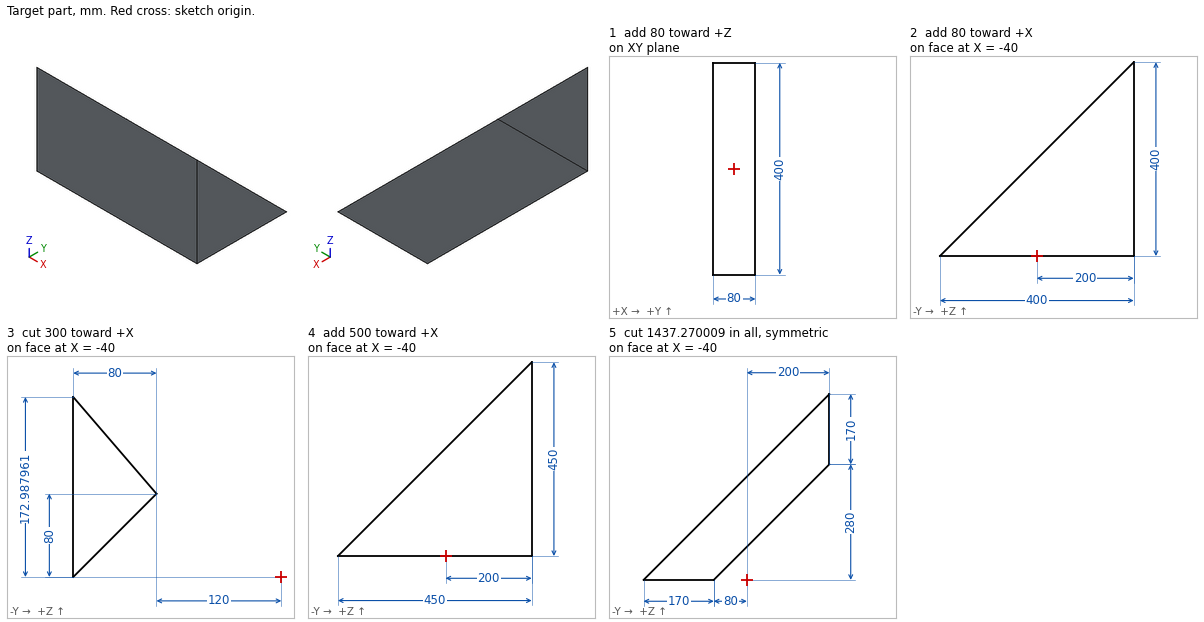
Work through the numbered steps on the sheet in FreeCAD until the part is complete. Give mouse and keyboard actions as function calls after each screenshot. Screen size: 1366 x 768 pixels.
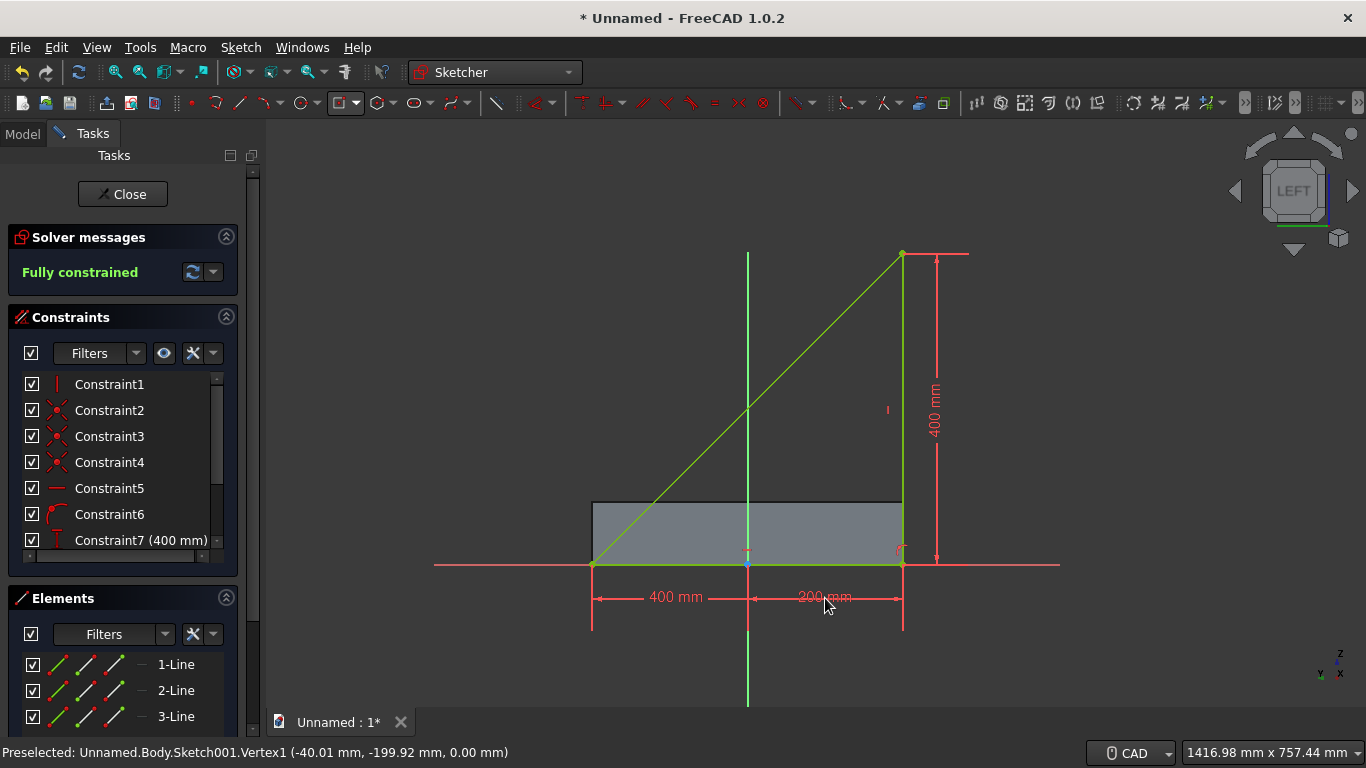
click(123, 194)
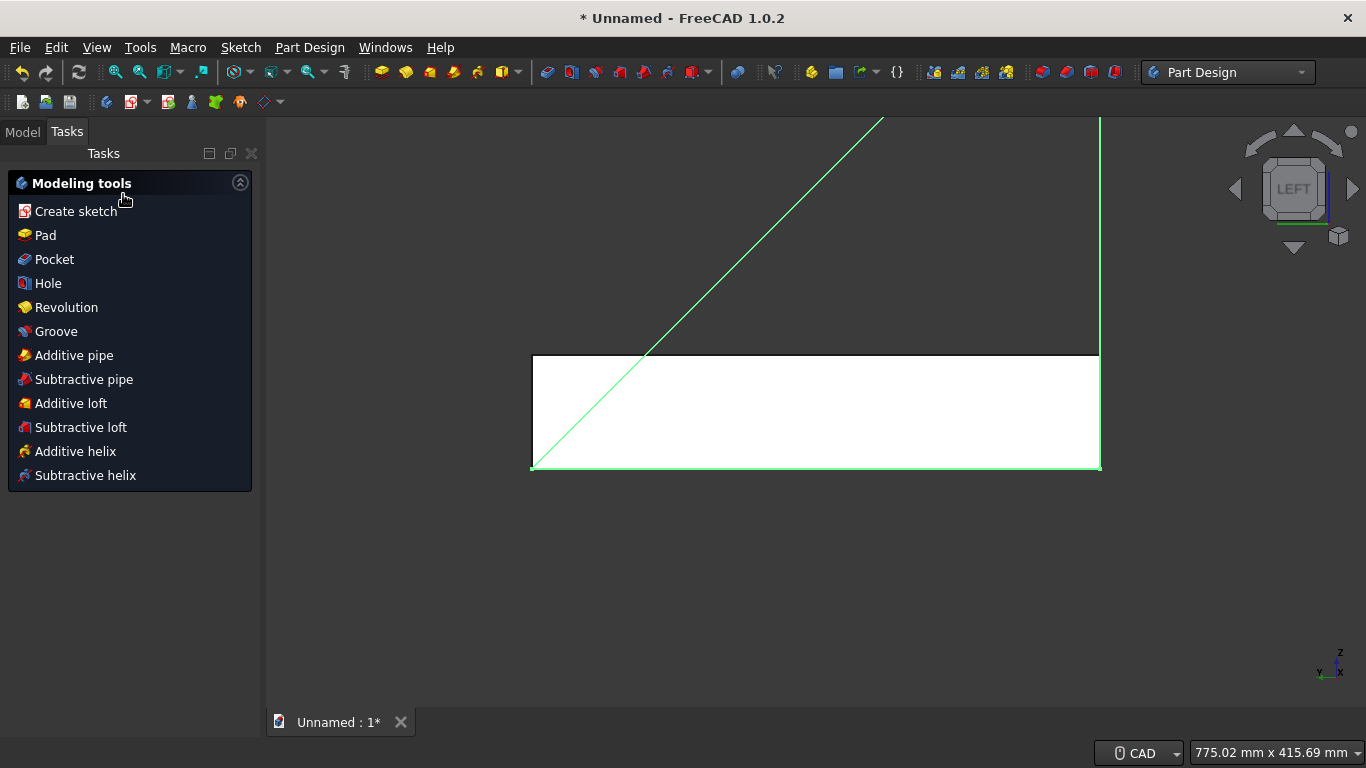
click(382, 72)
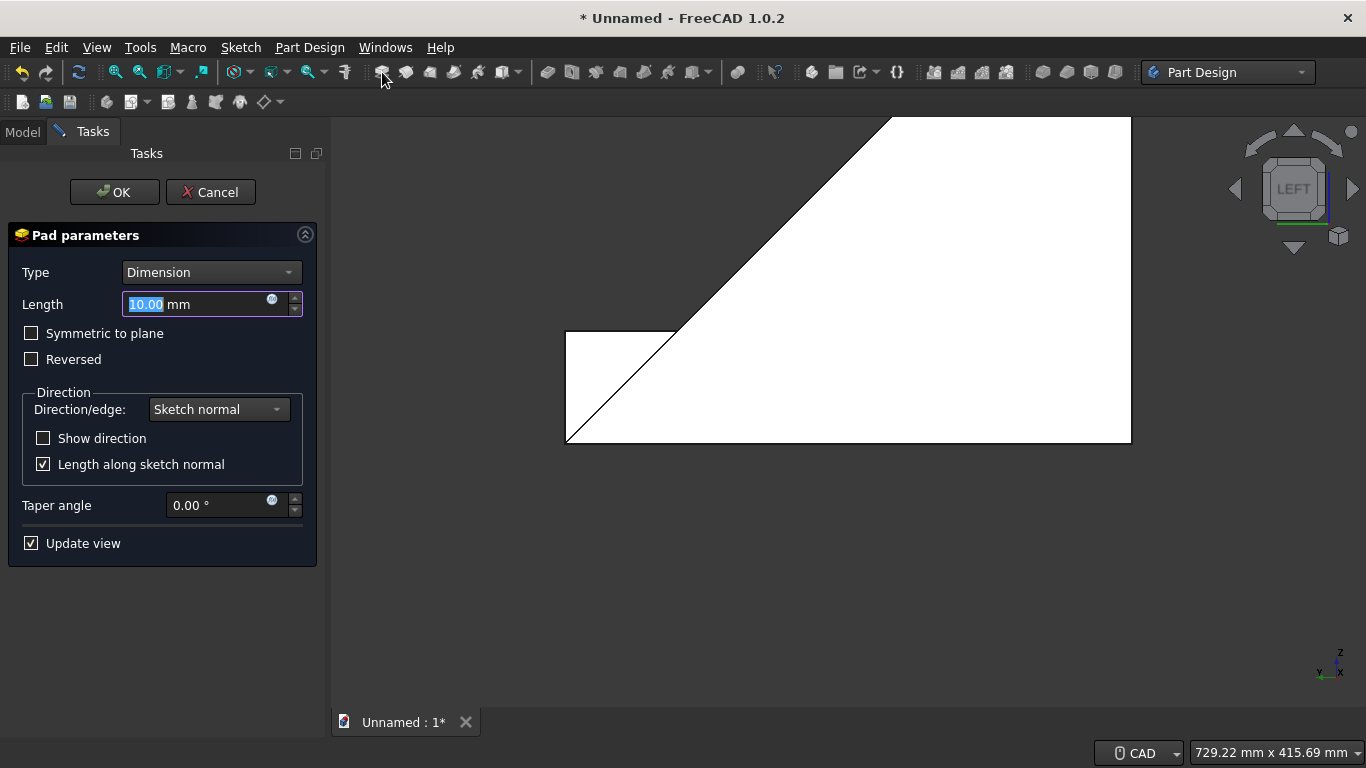
text(80)
key(Tab)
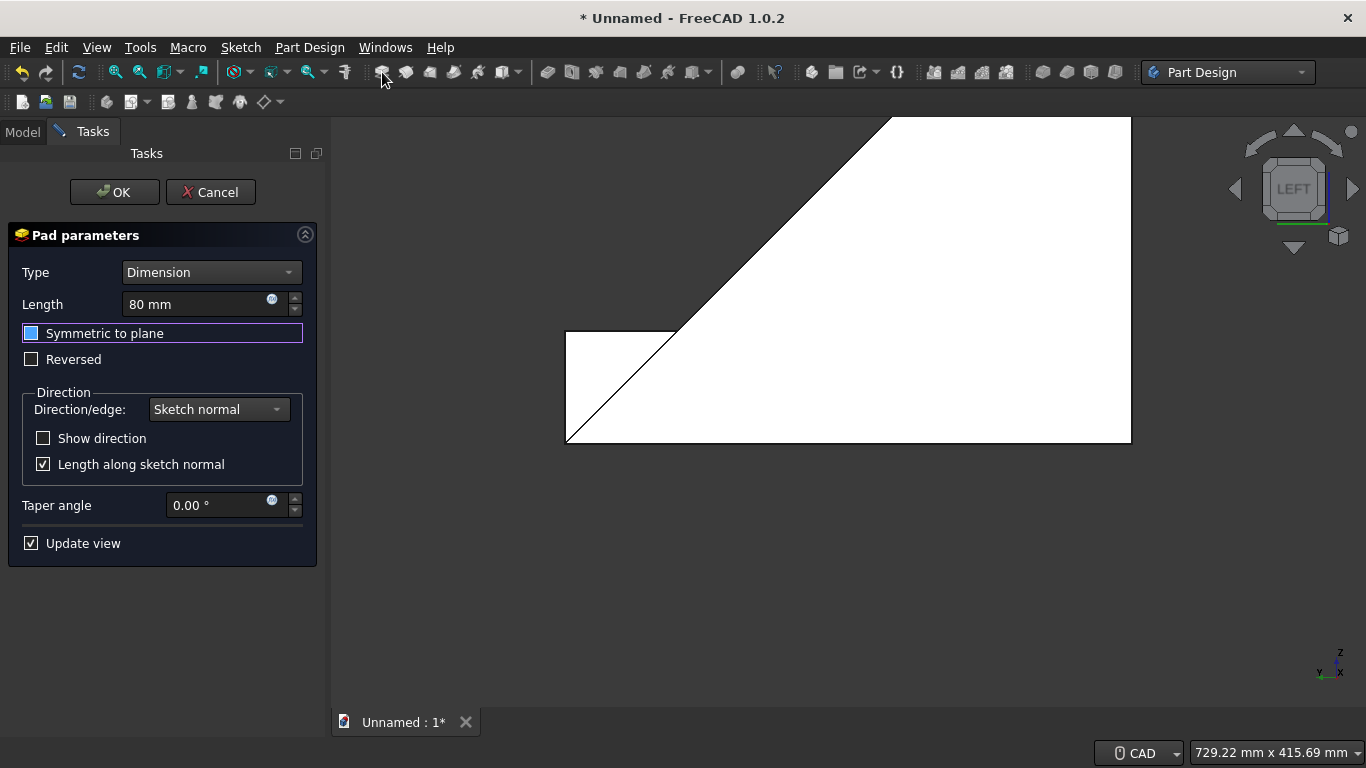
click(30, 359)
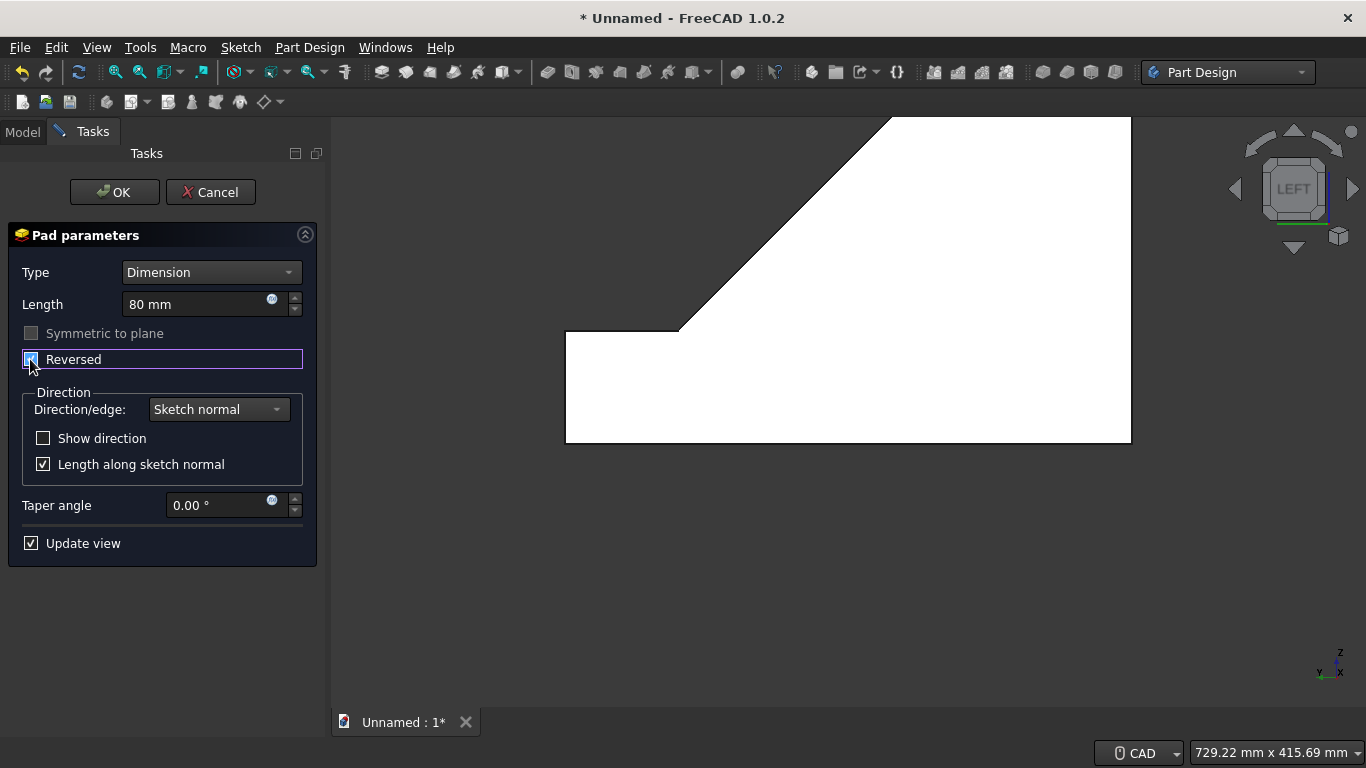
click(115, 192)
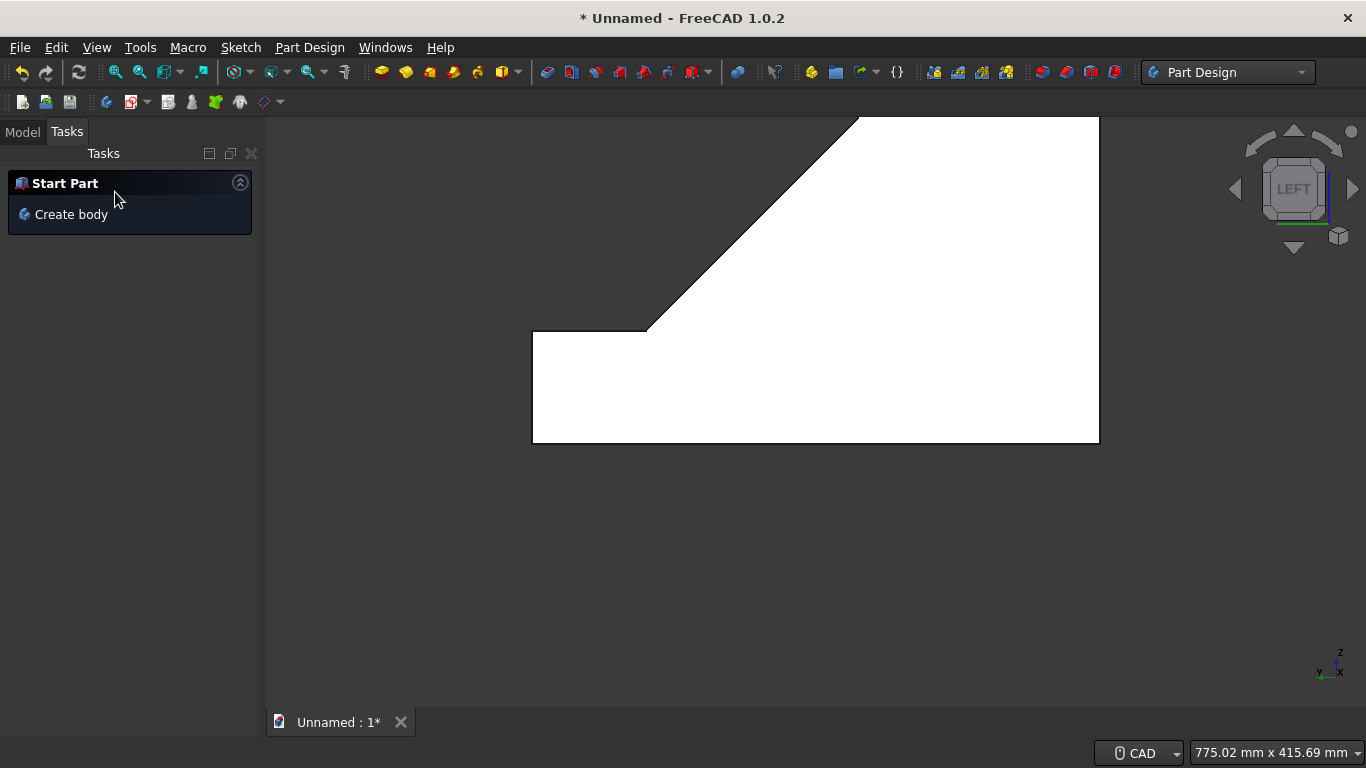
click(116, 72)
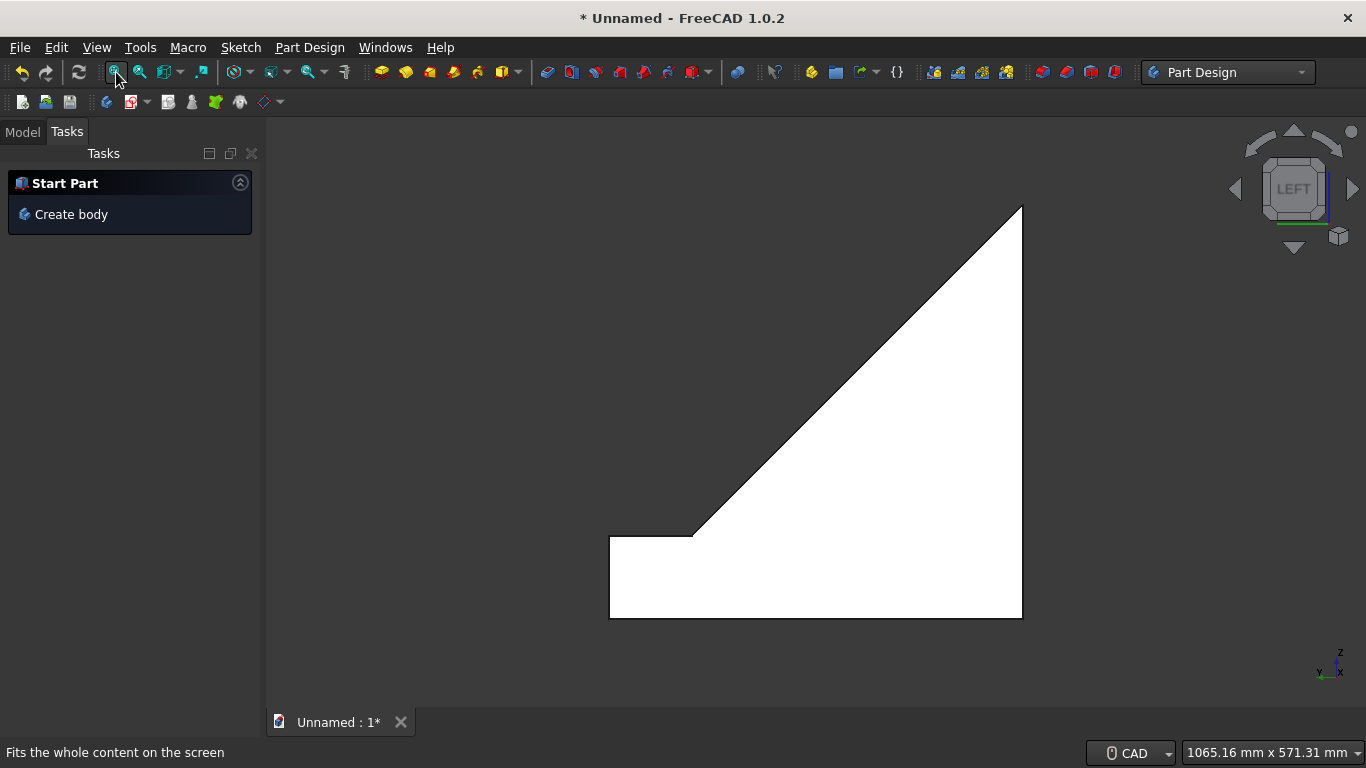
click(875, 529)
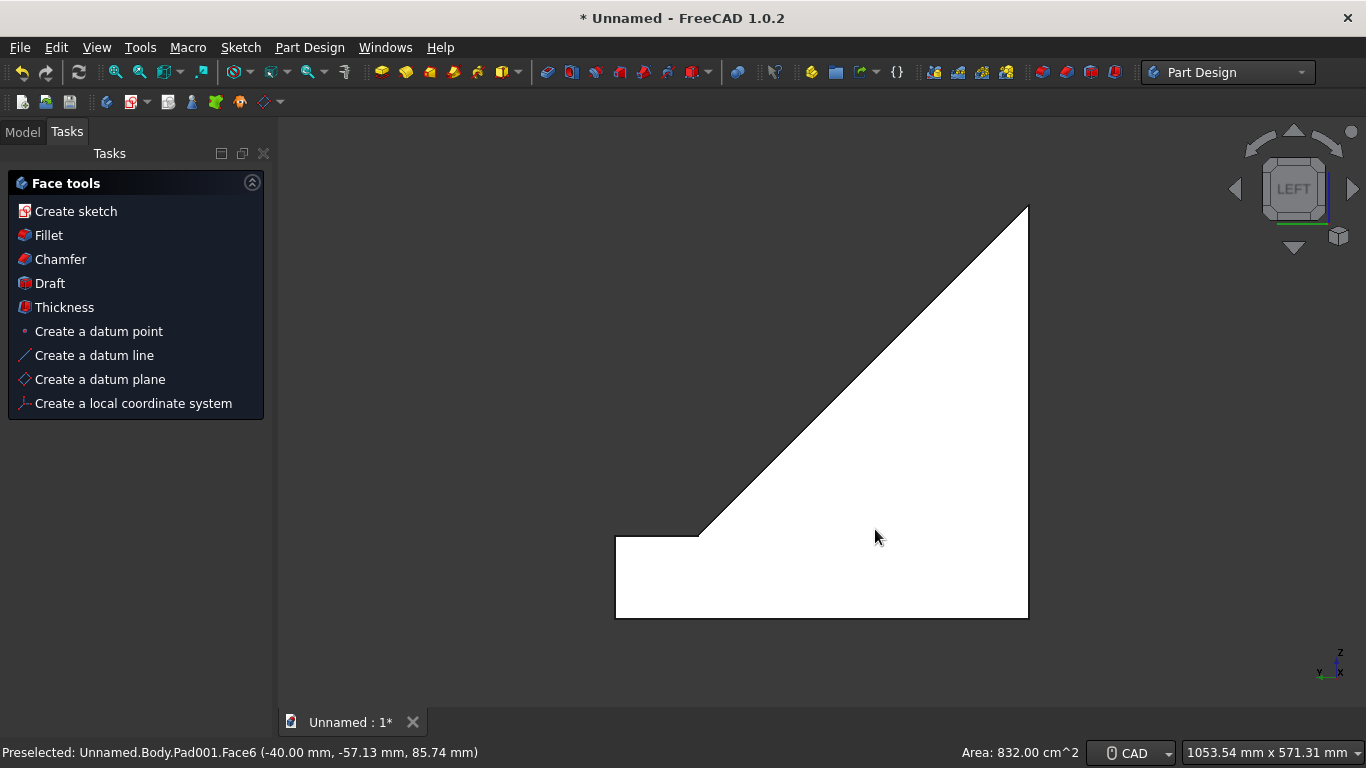
click(132, 102)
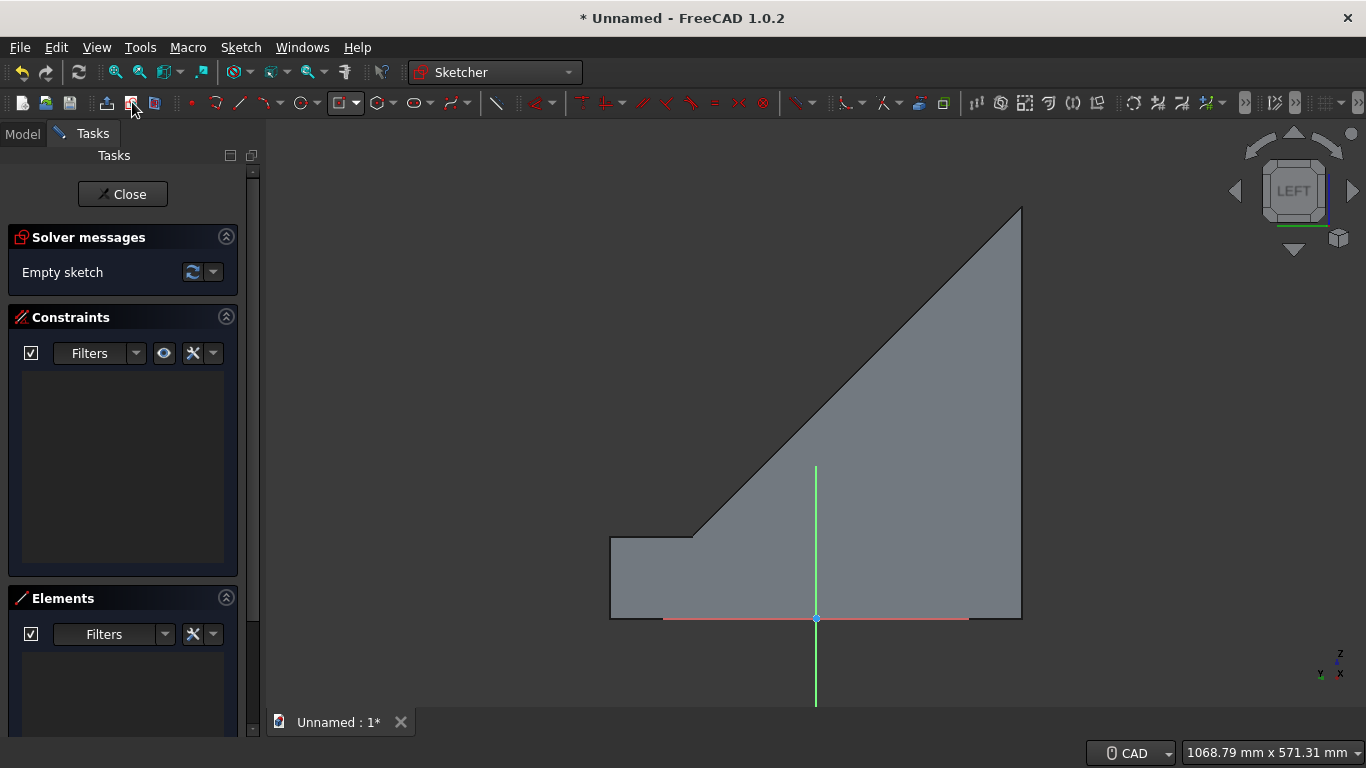
scroll(685, 625, up, 4)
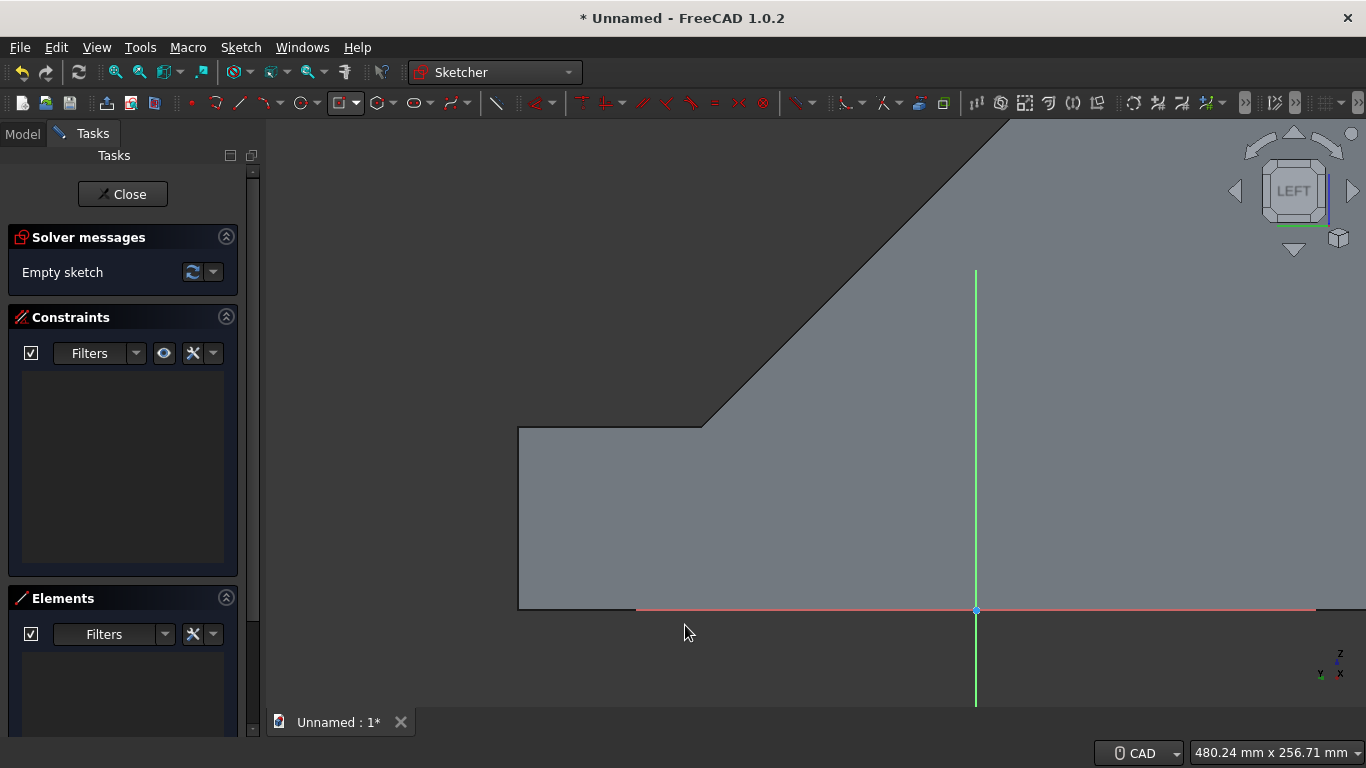
click(216, 104)